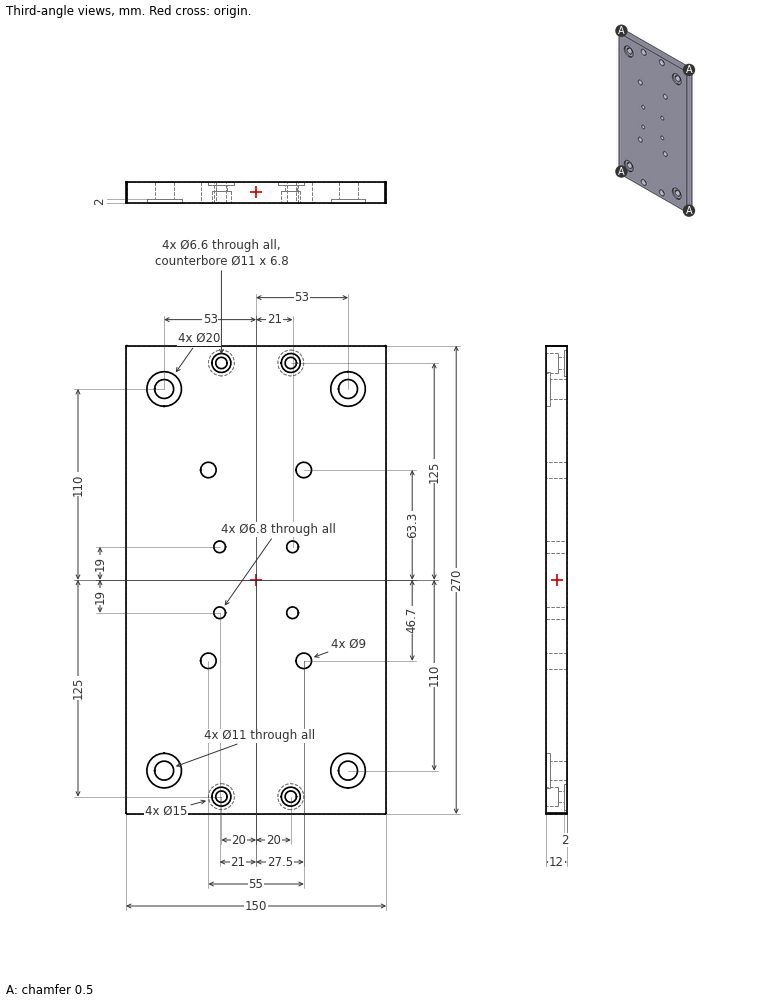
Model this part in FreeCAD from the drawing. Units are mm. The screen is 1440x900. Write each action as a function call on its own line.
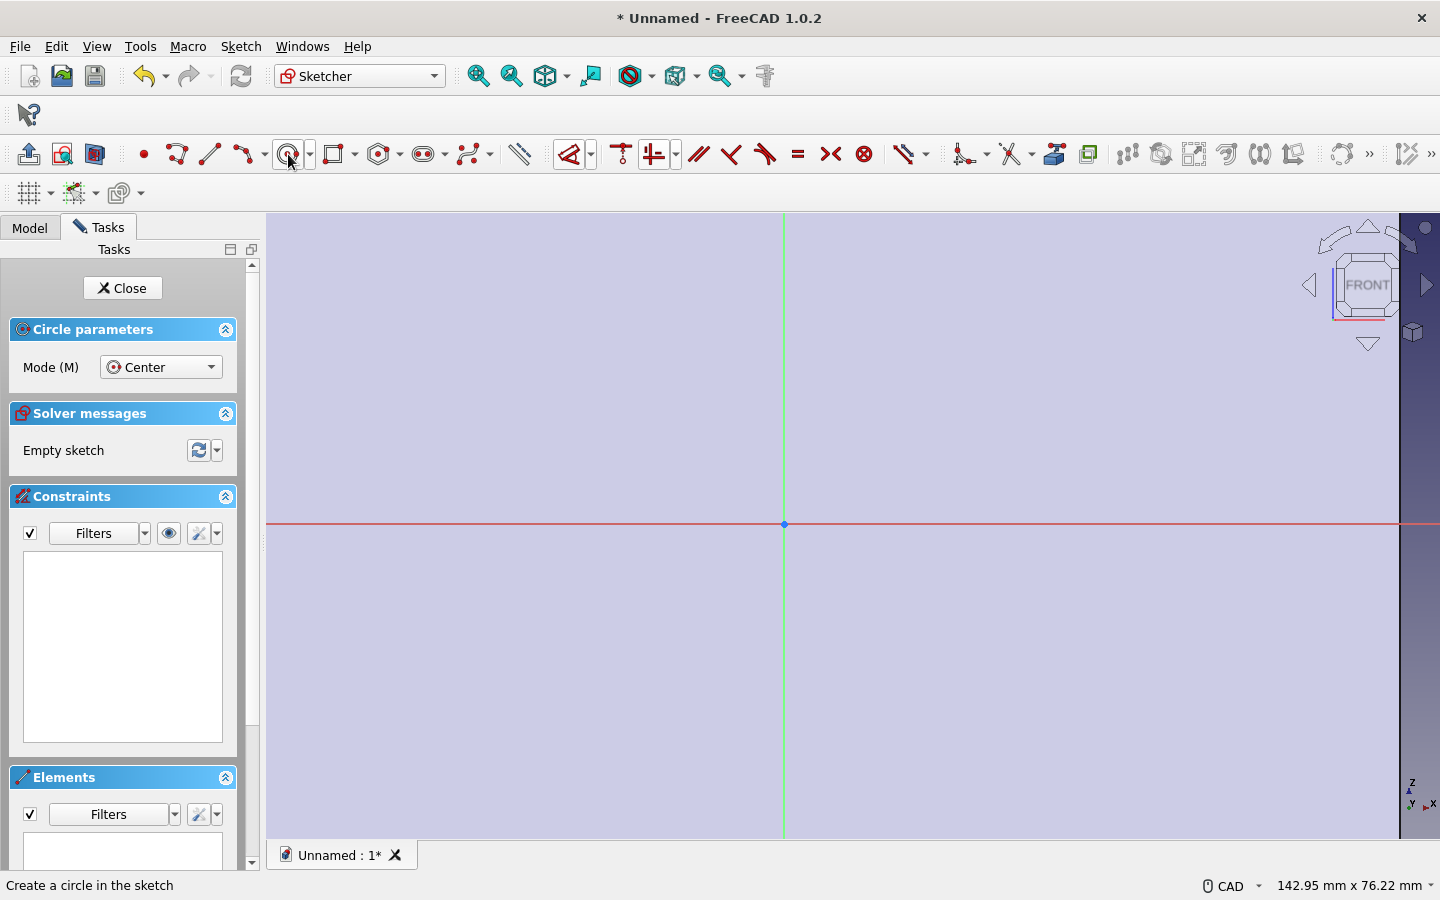
click(612, 681)
click(631, 661)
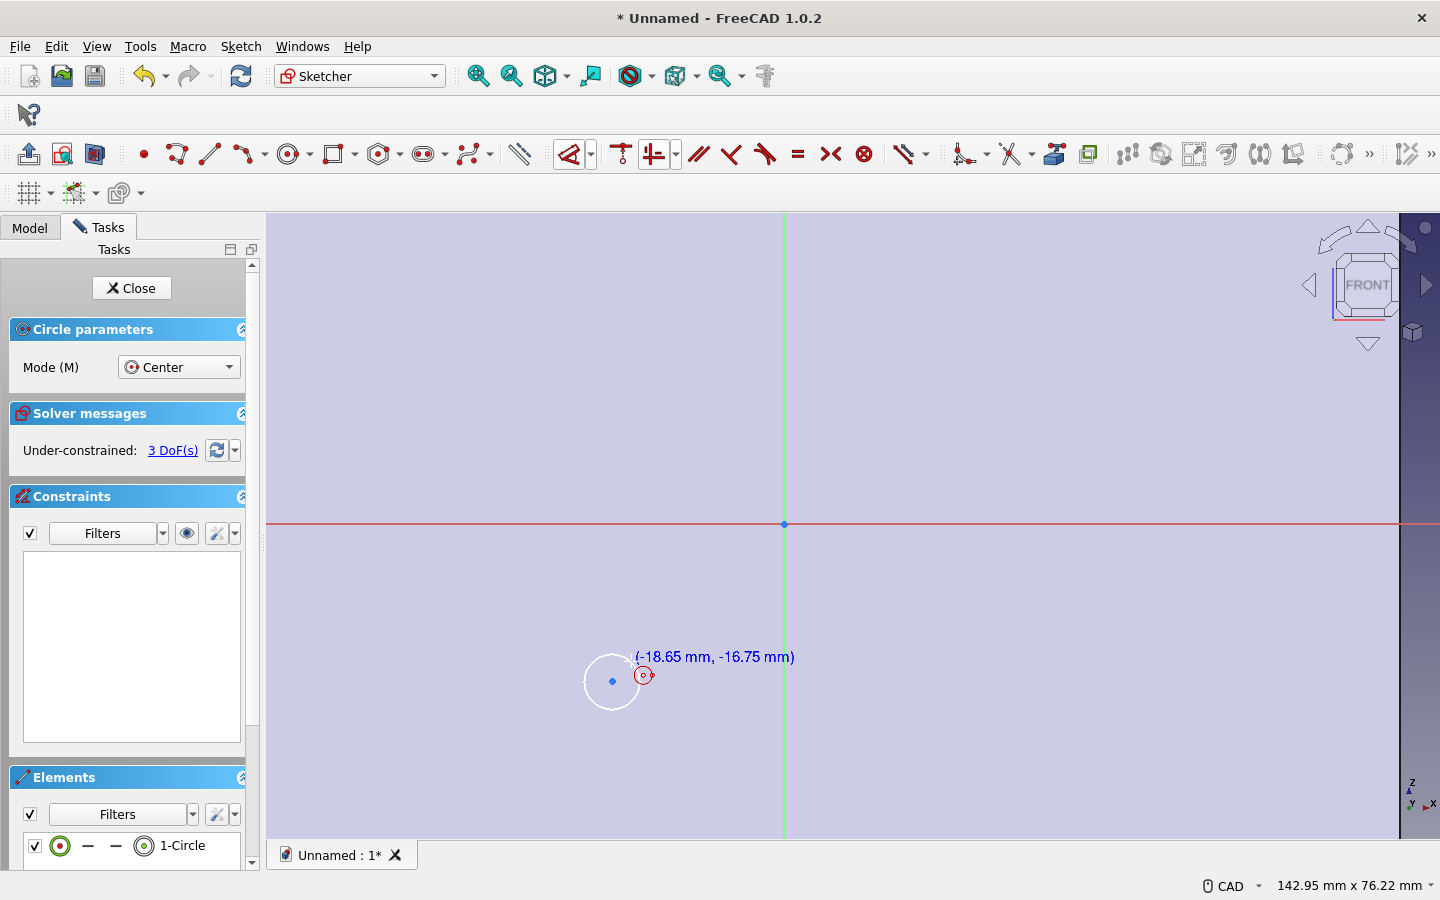
click(612, 368)
click(631, 349)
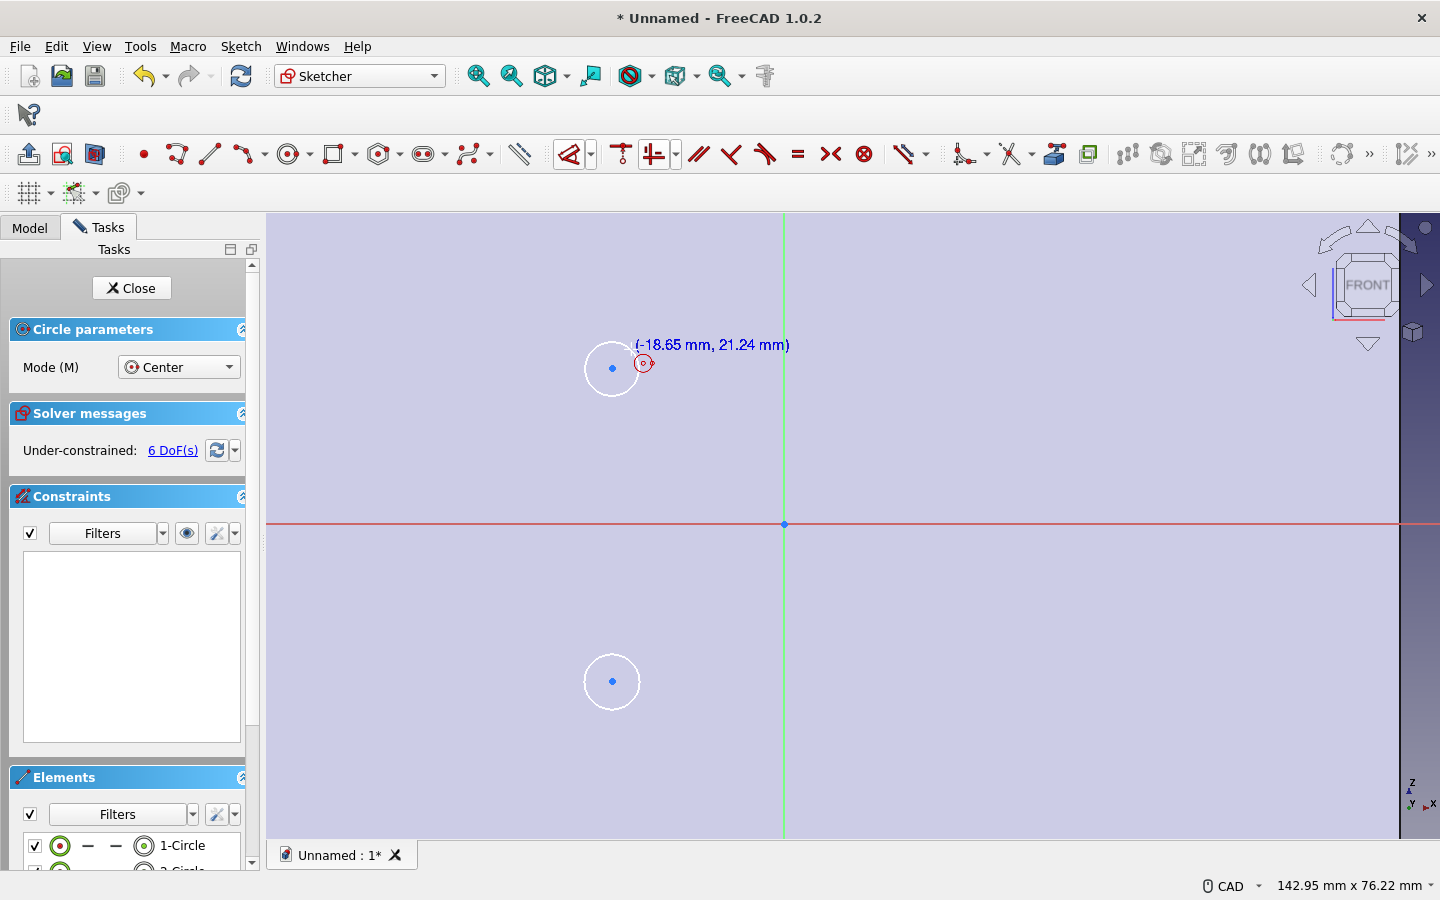
click(957, 368)
click(976, 349)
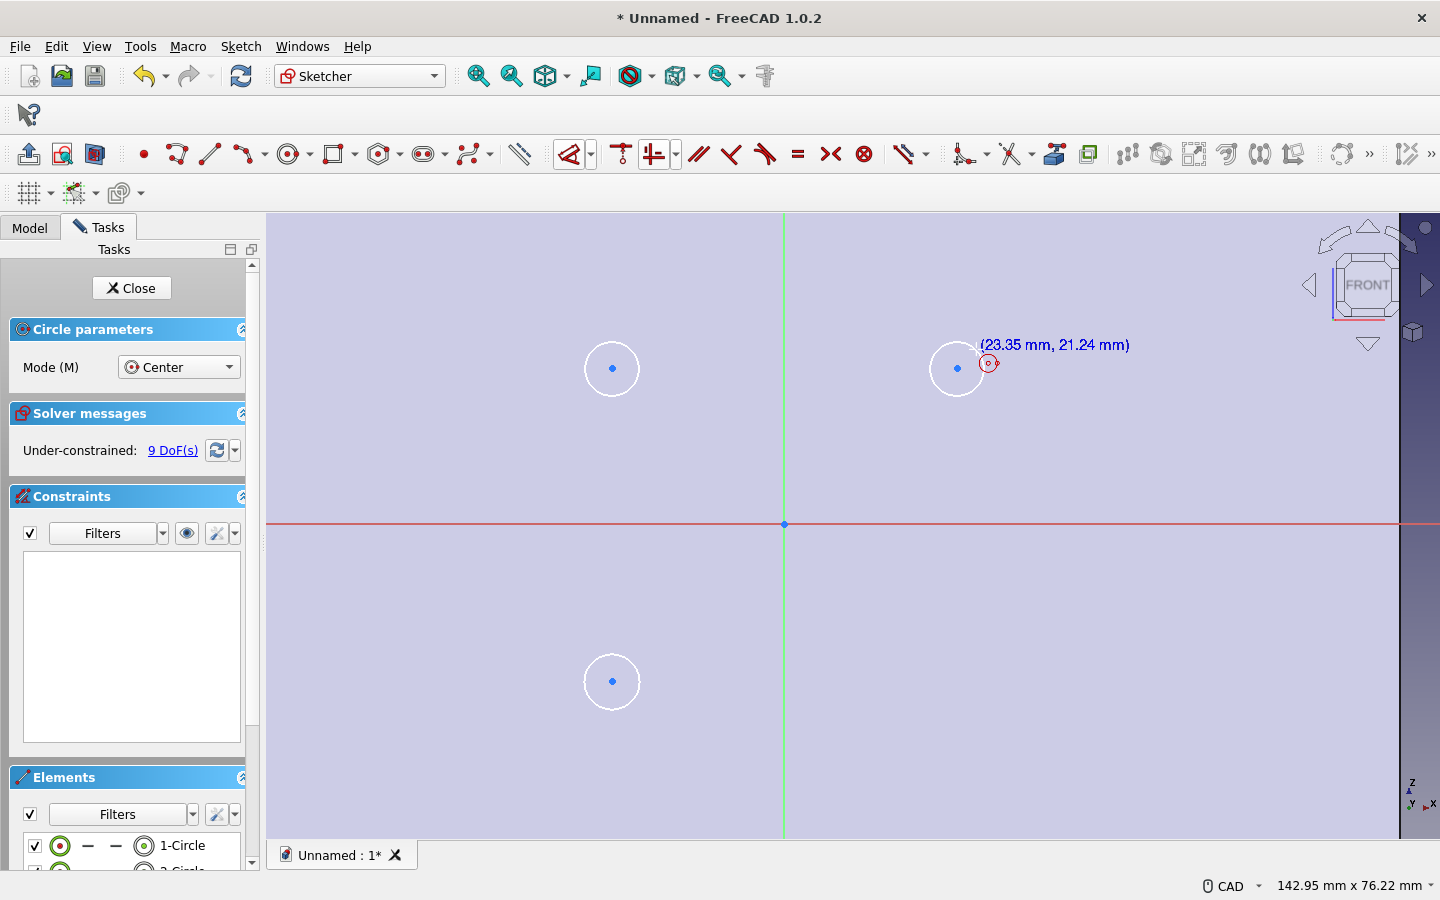
click(957, 681)
click(976, 661)
key(Escape)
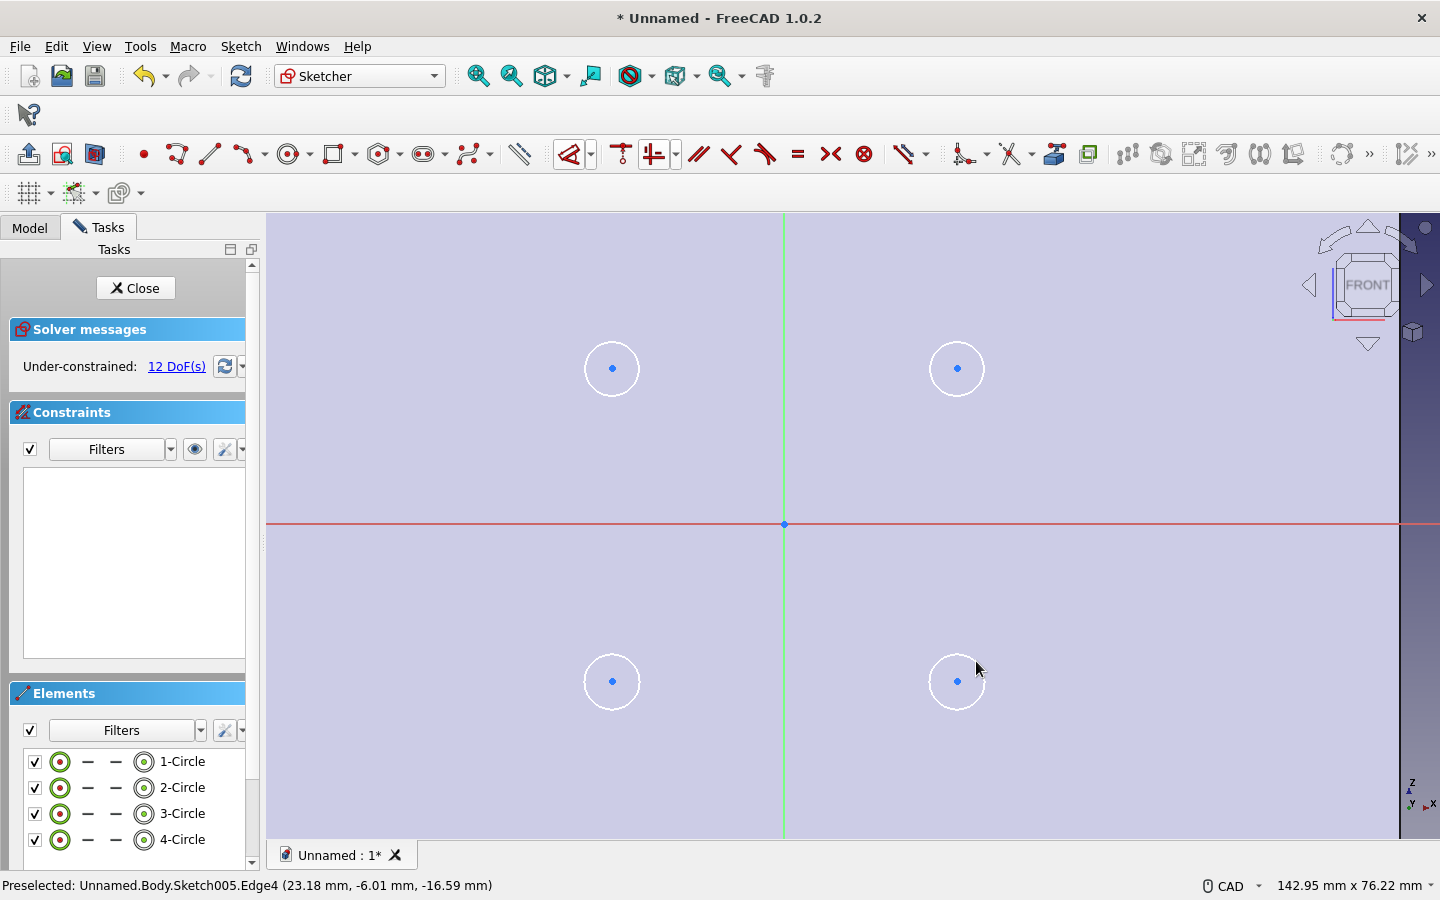
click(631, 662)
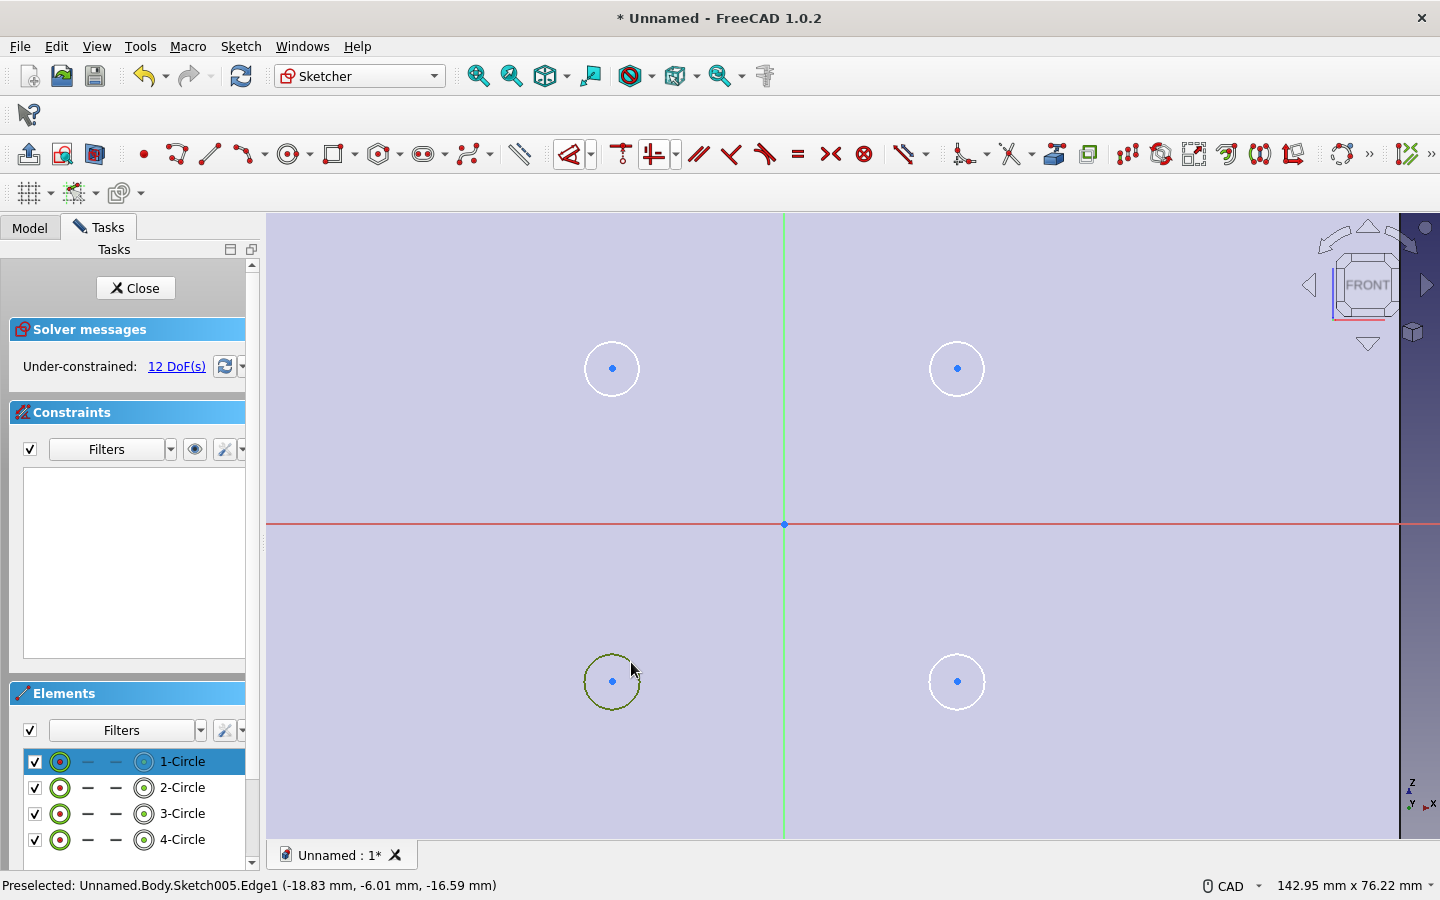
click(631, 350)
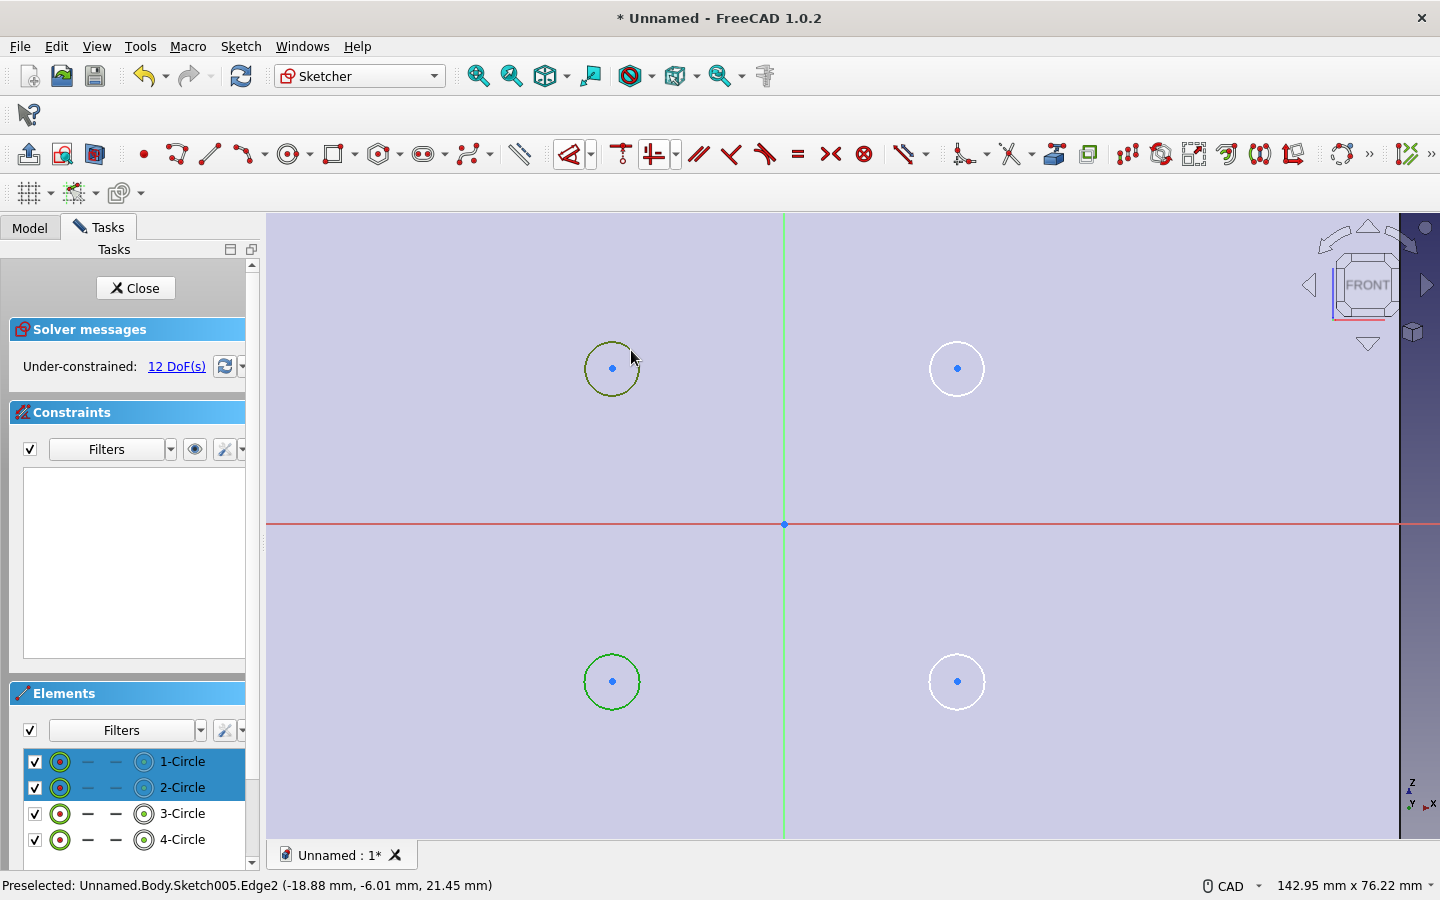
click(976, 350)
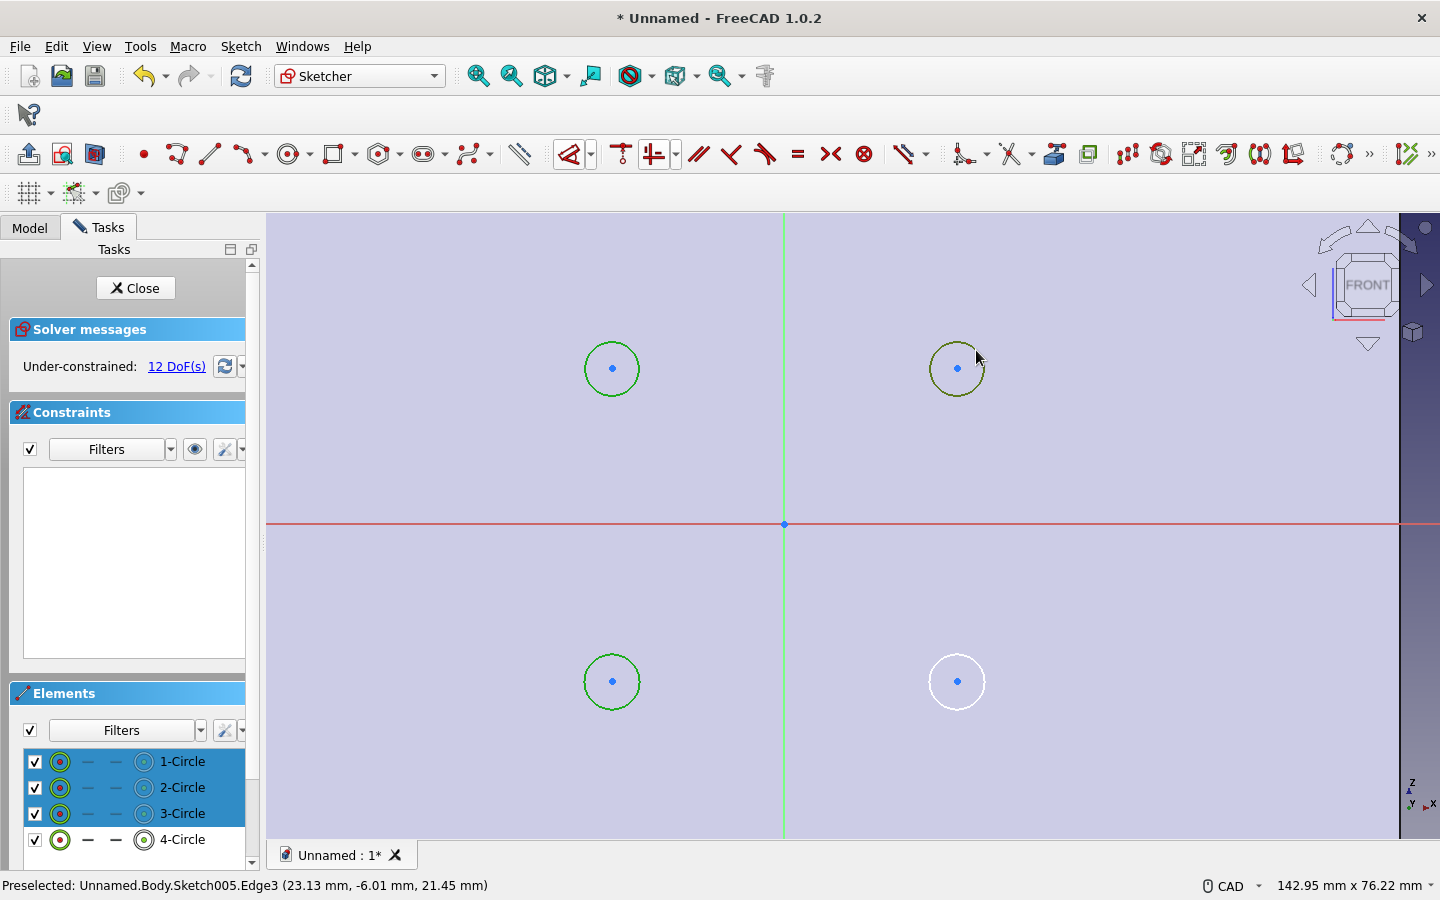
click(976, 662)